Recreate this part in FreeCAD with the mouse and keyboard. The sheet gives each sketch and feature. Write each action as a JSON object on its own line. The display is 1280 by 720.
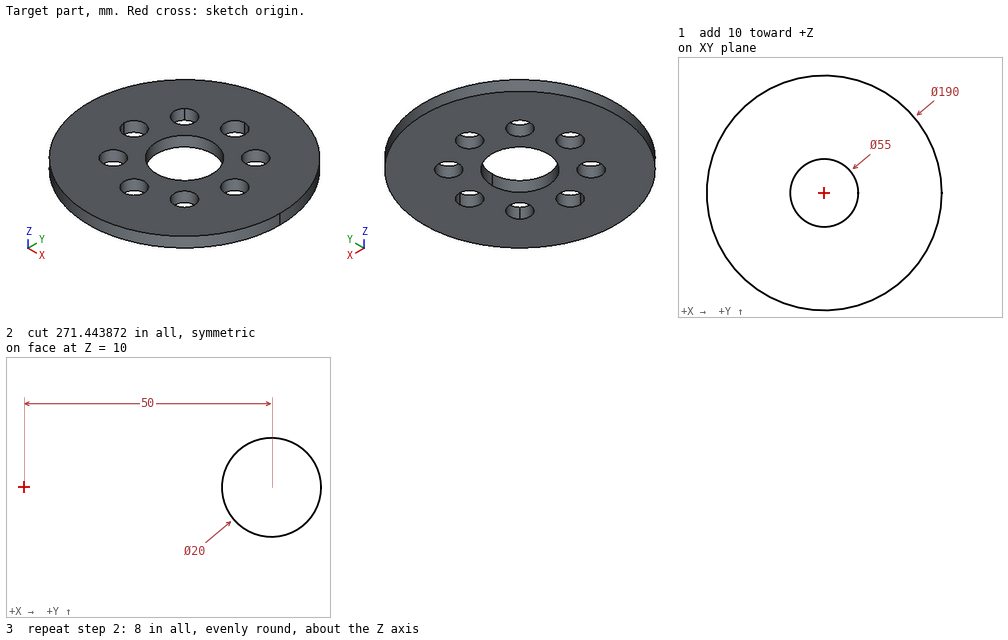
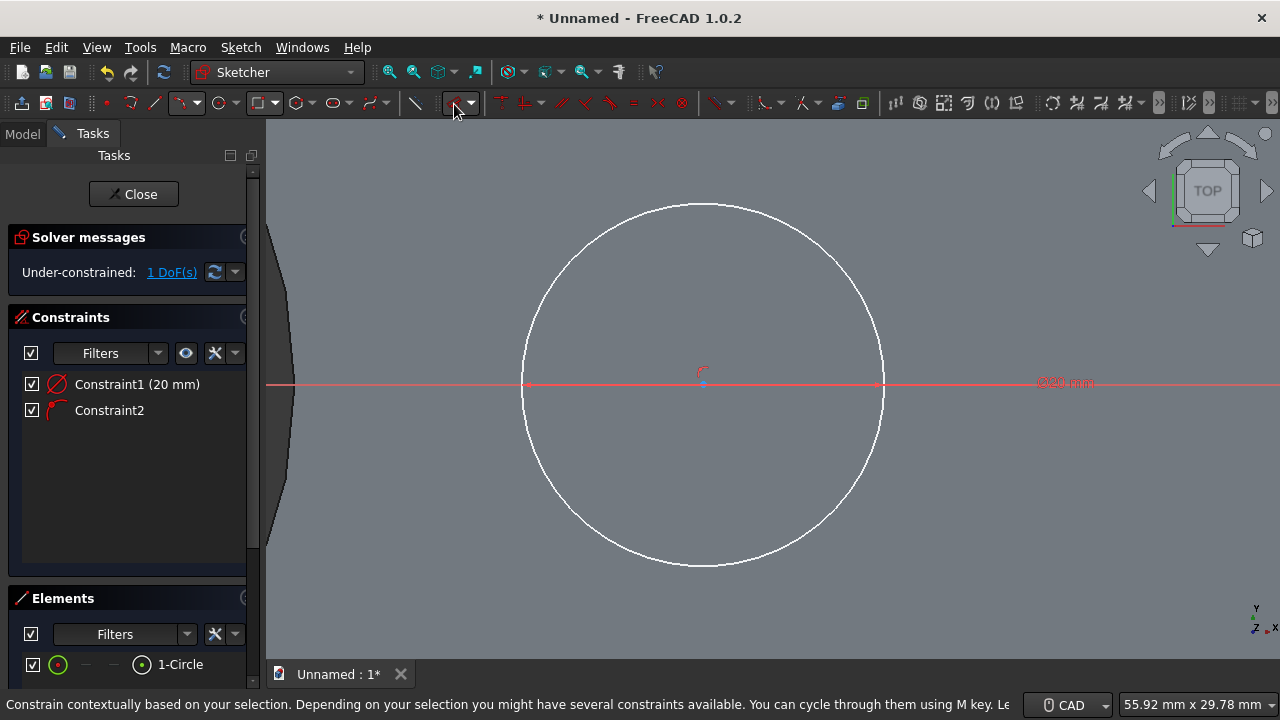
{"action": "left_click", "coordinate": [703, 385]}
{"action": "left_click", "coordinate": [498, 419]}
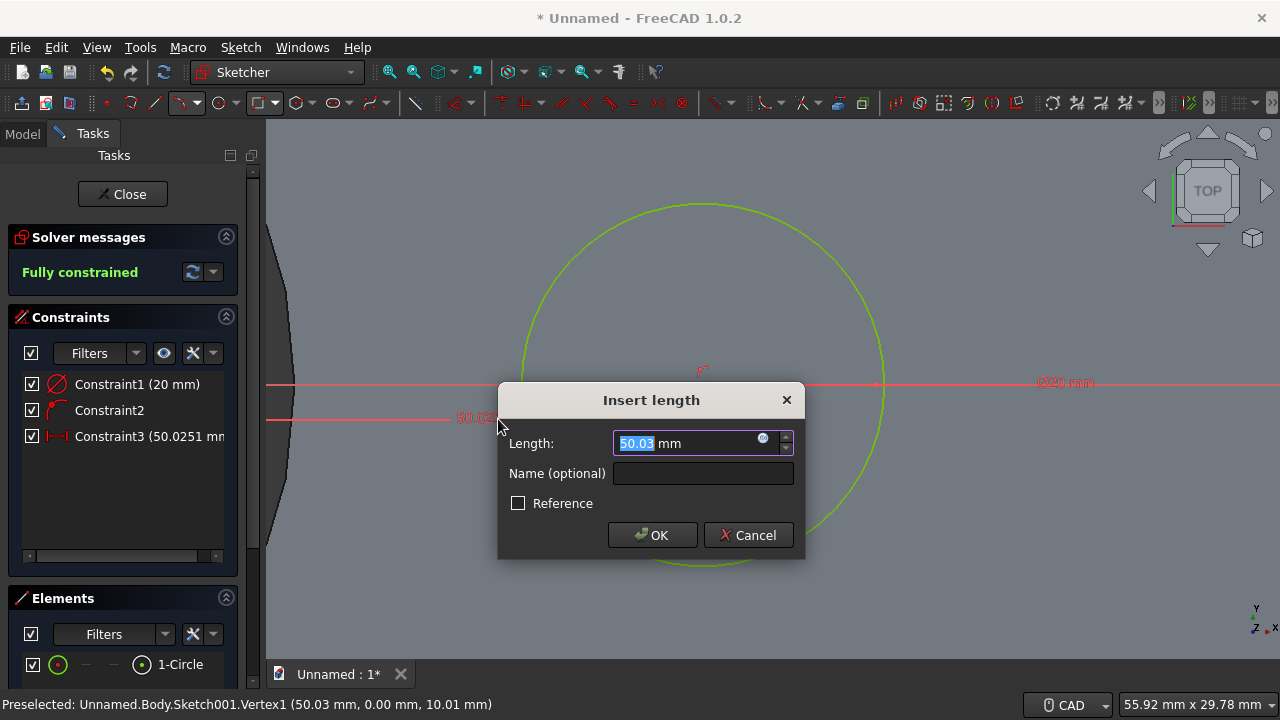
{"action": "type", "text": "50"}
{"action": "key", "text": "Return"}
{"action": "key", "text": "Escape"}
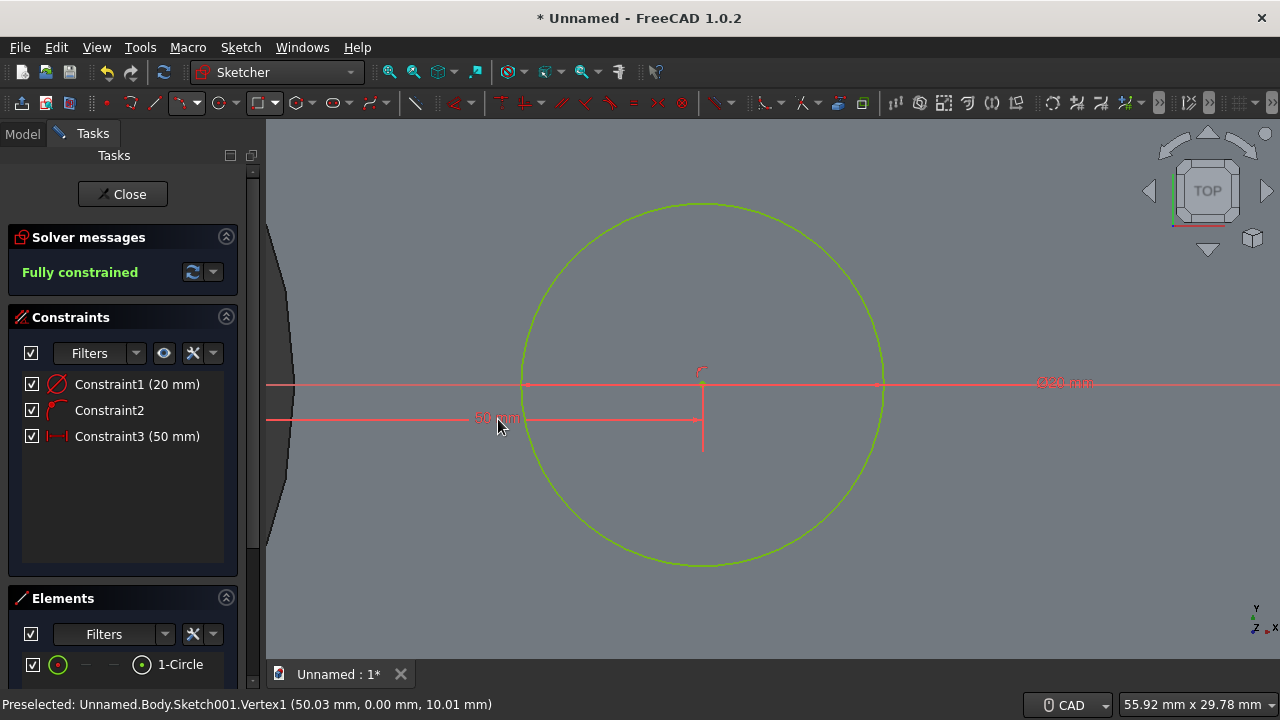
{"action": "left_click", "coordinate": [123, 194]}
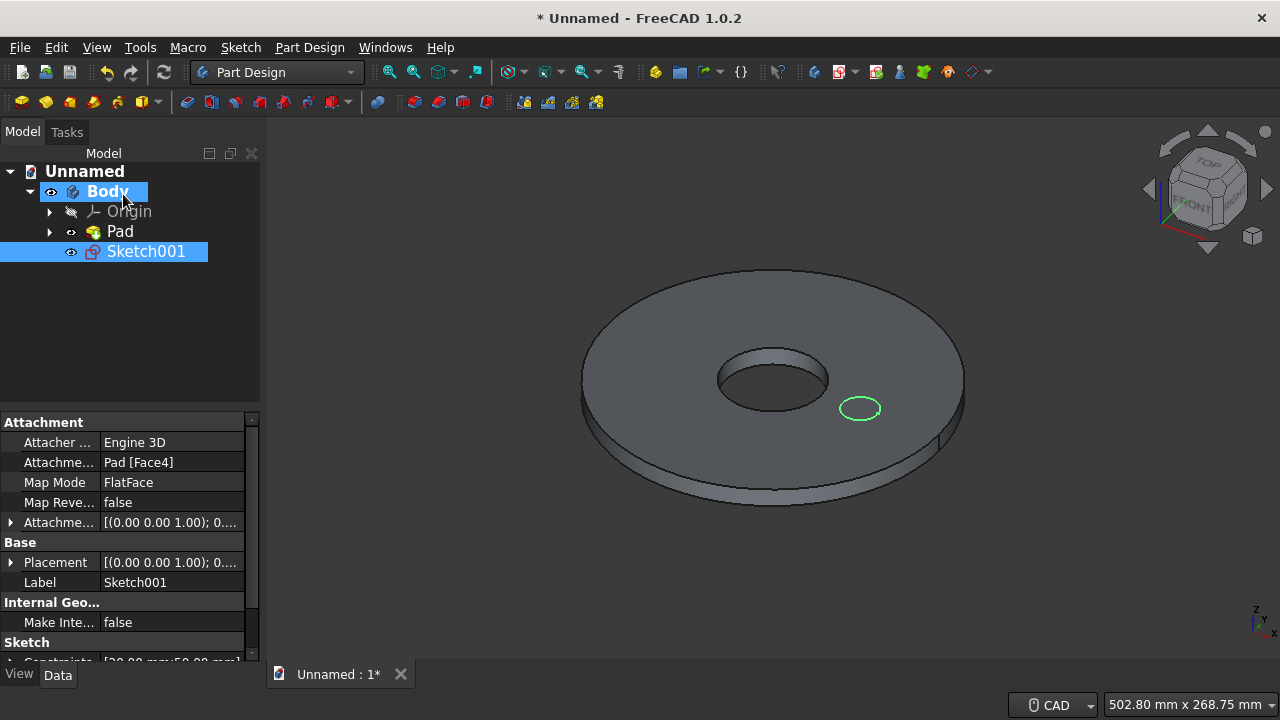
{"action": "left_click", "coordinate": [188, 102]}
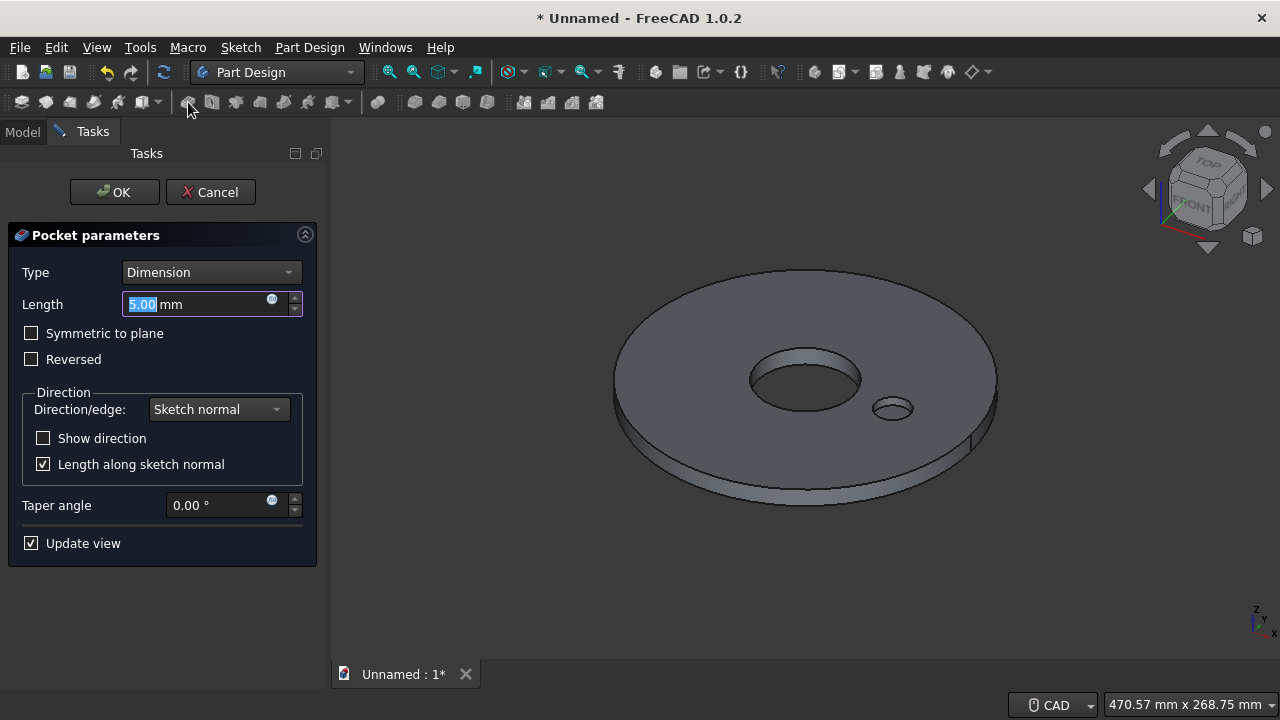
{"action": "type", "text": "271.443872"}
{"action": "key", "text": "Tab"}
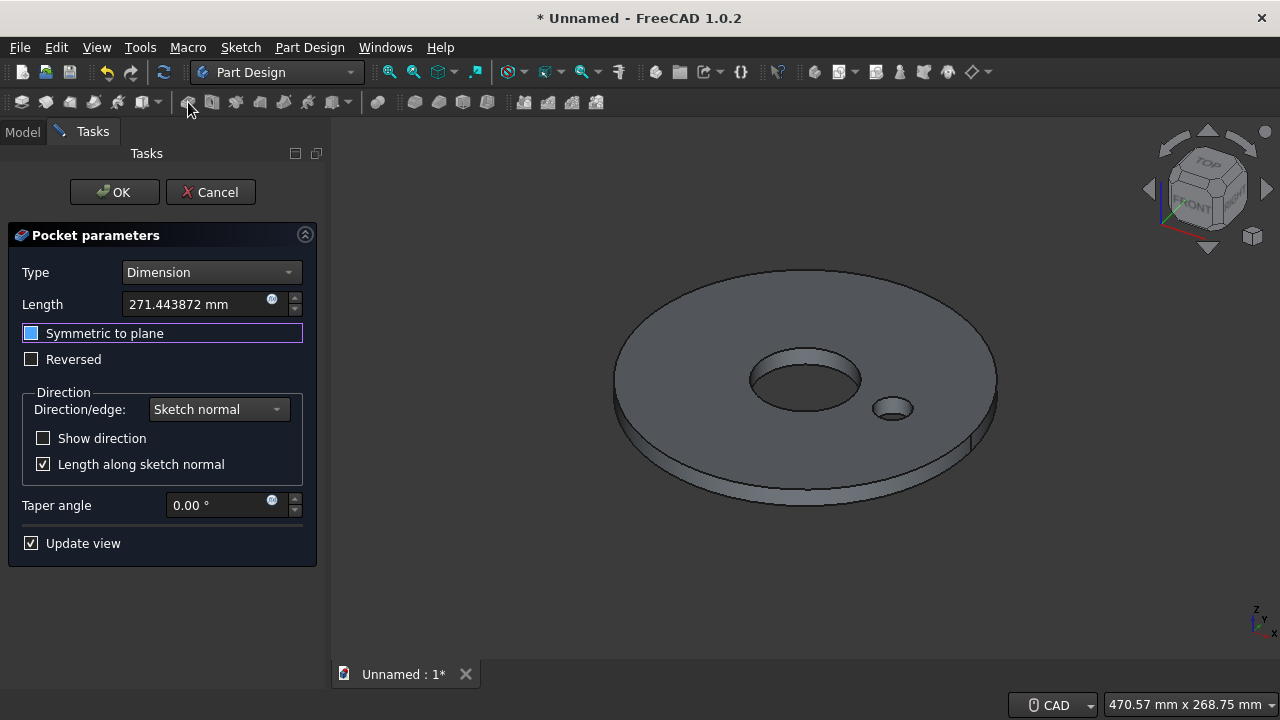
{"action": "left_click", "coordinate": [30, 333]}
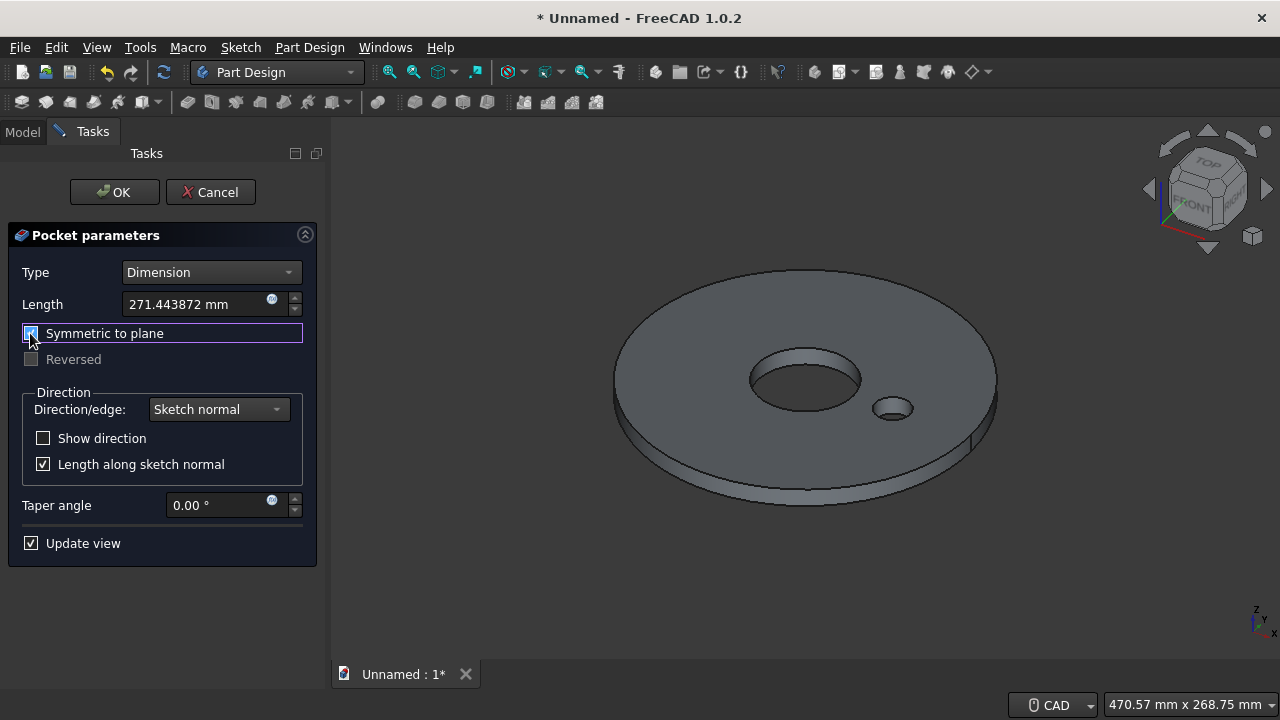
{"action": "left_click", "coordinate": [115, 192]}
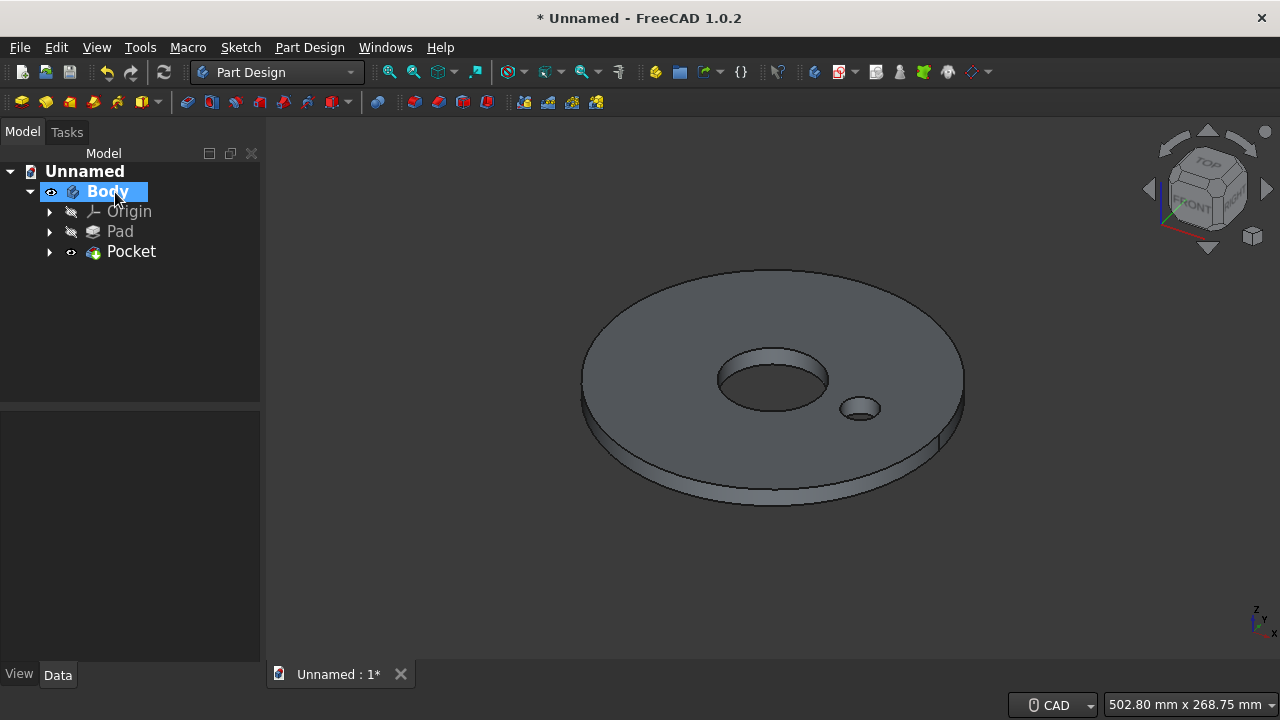
{"action": "left_click", "coordinate": [116, 252]}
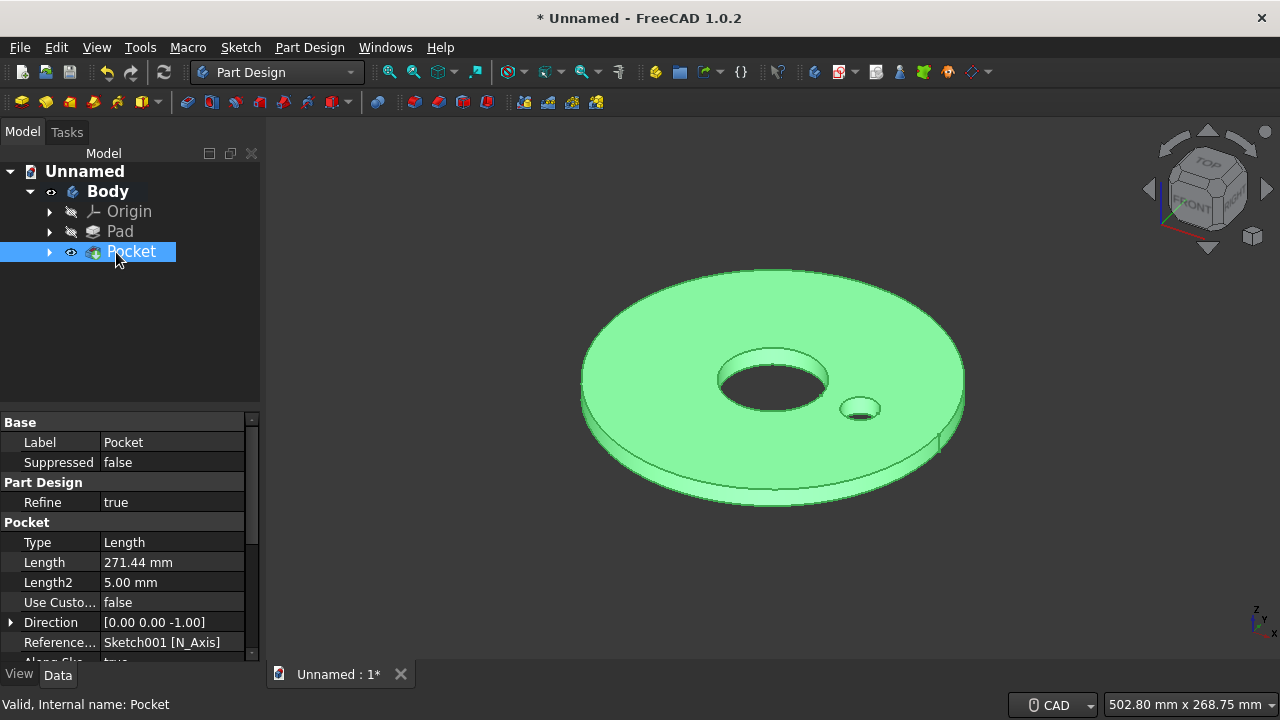
{"action": "left_click", "coordinate": [572, 102]}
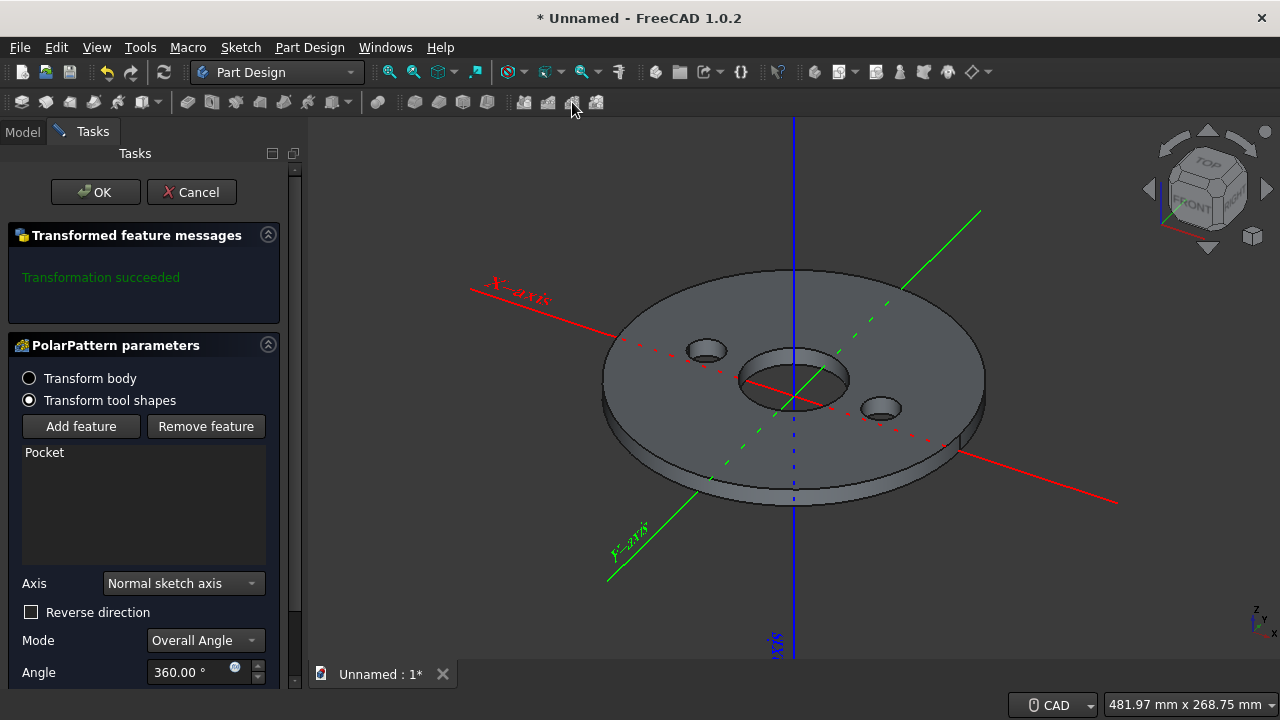
{"action": "left_click", "coordinate": [184, 584]}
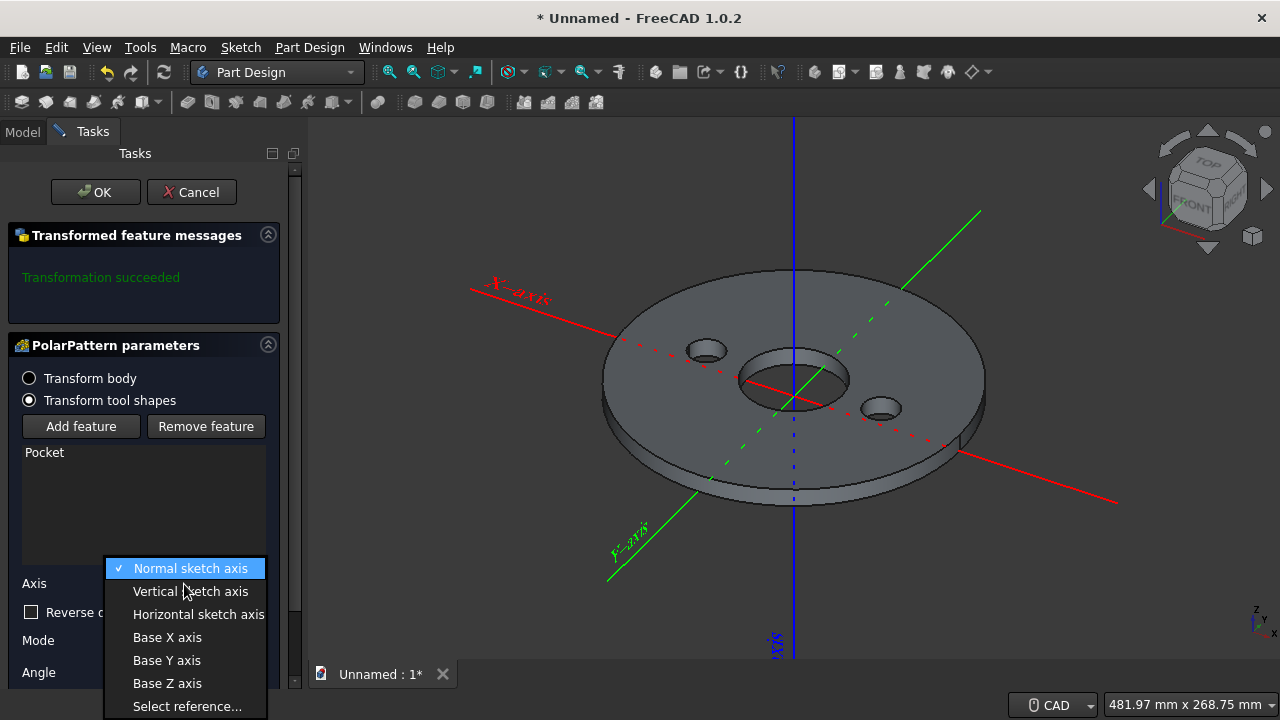
{"action": "left_click", "coordinate": [184, 684]}